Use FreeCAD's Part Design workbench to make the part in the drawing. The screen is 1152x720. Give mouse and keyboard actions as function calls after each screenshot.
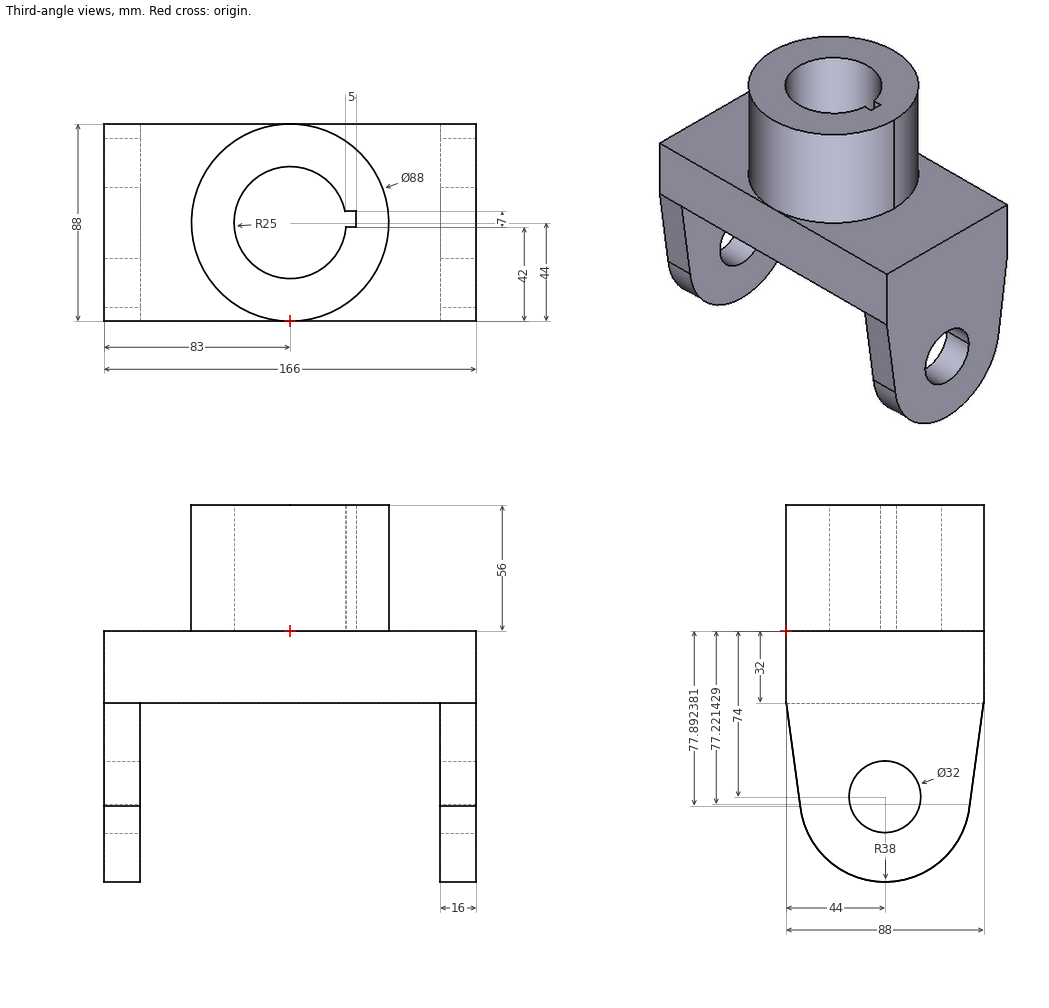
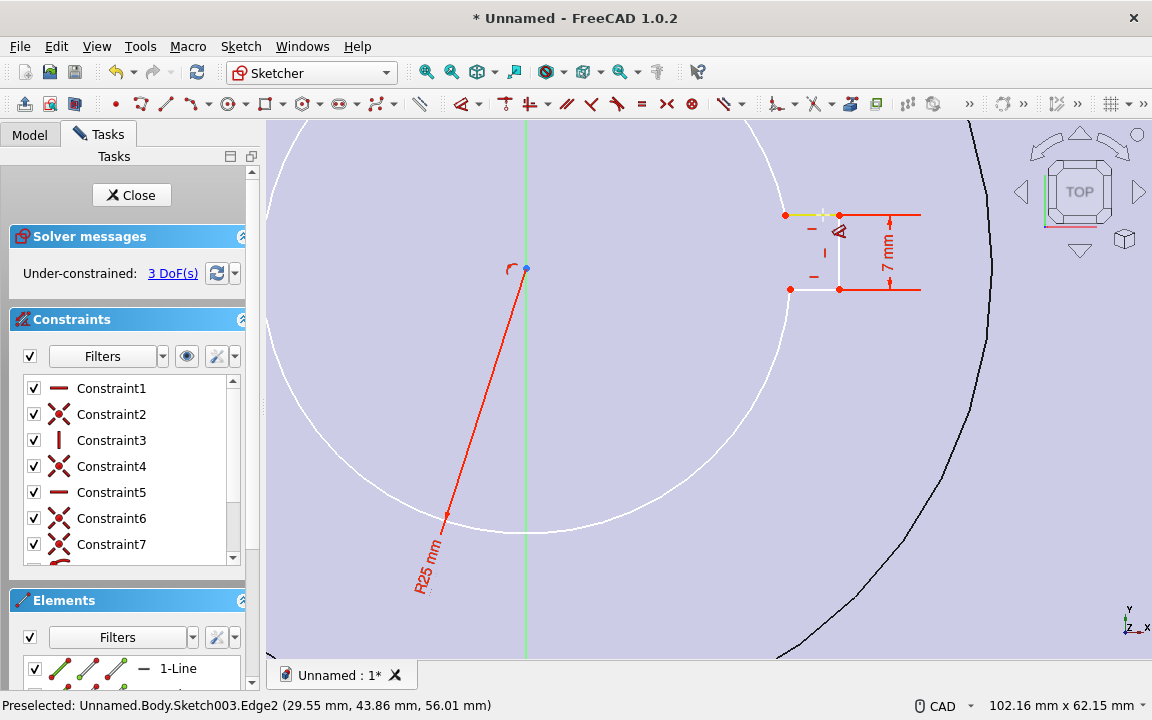
click(823, 215)
click(812, 181)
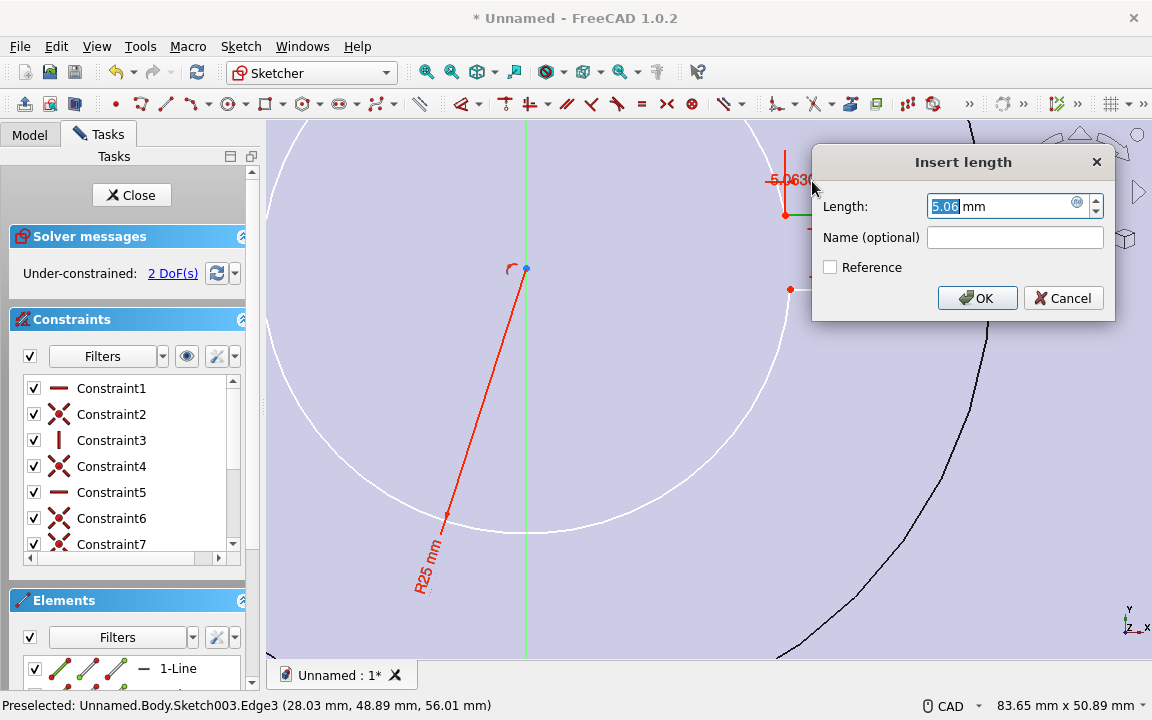
text(5)
key(Return)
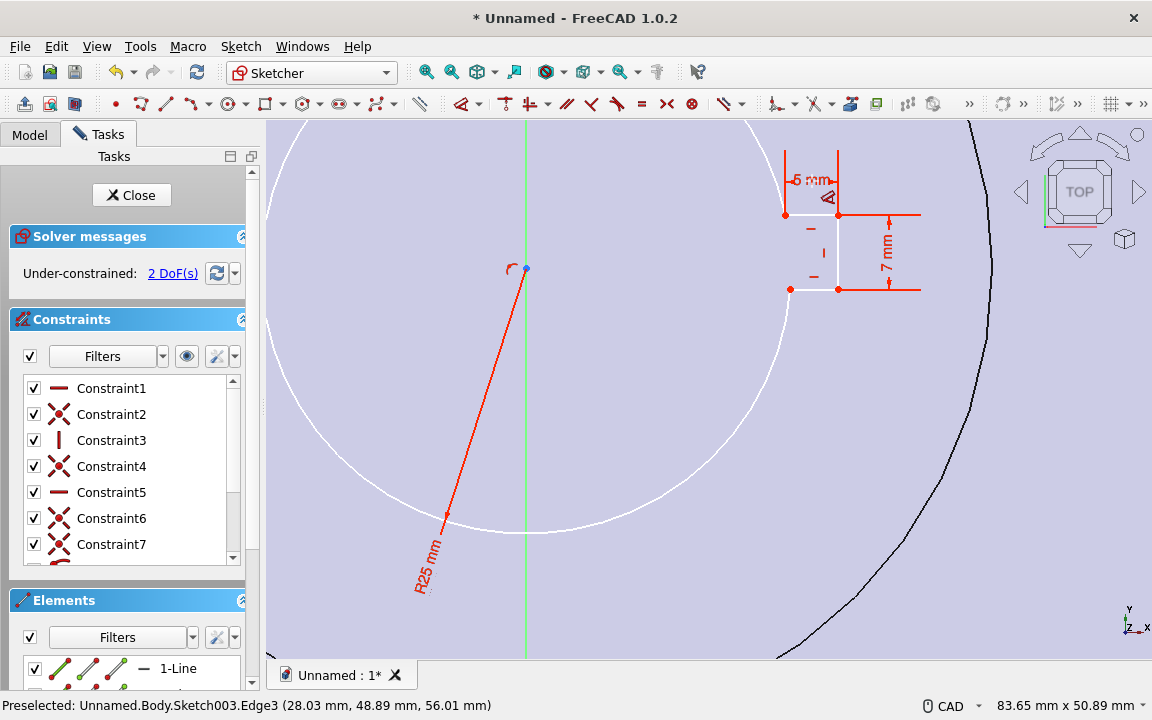
click(790, 290)
click(824, 460)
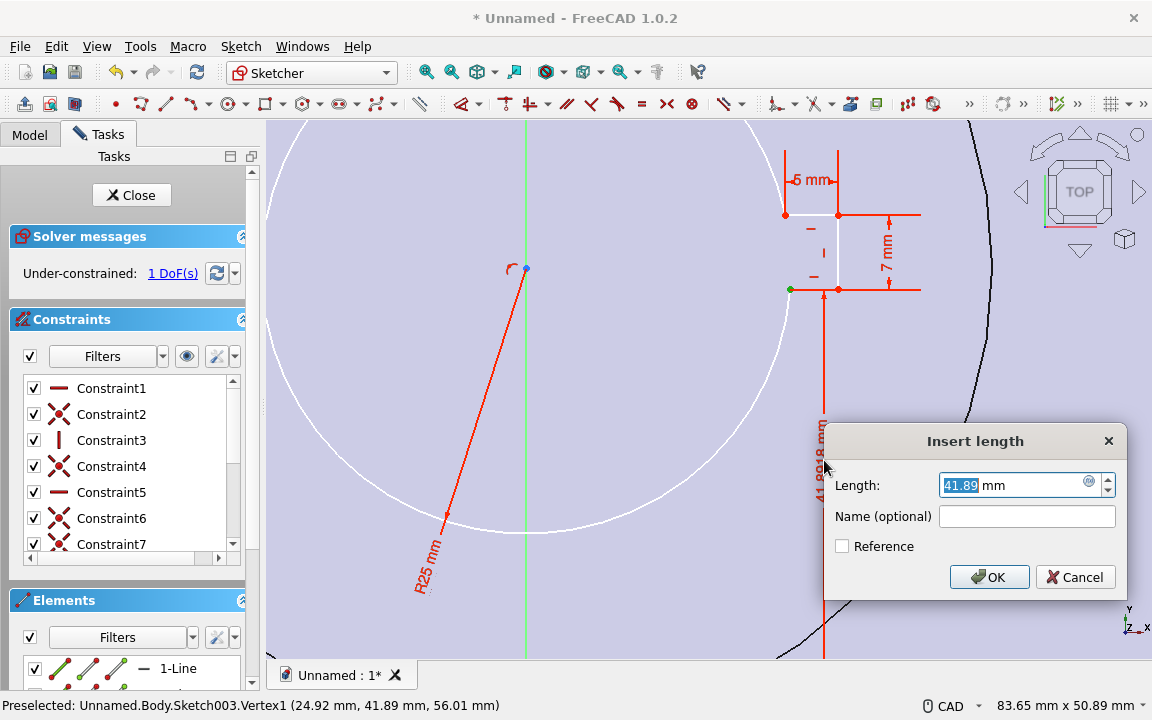
text(42)
key(Return)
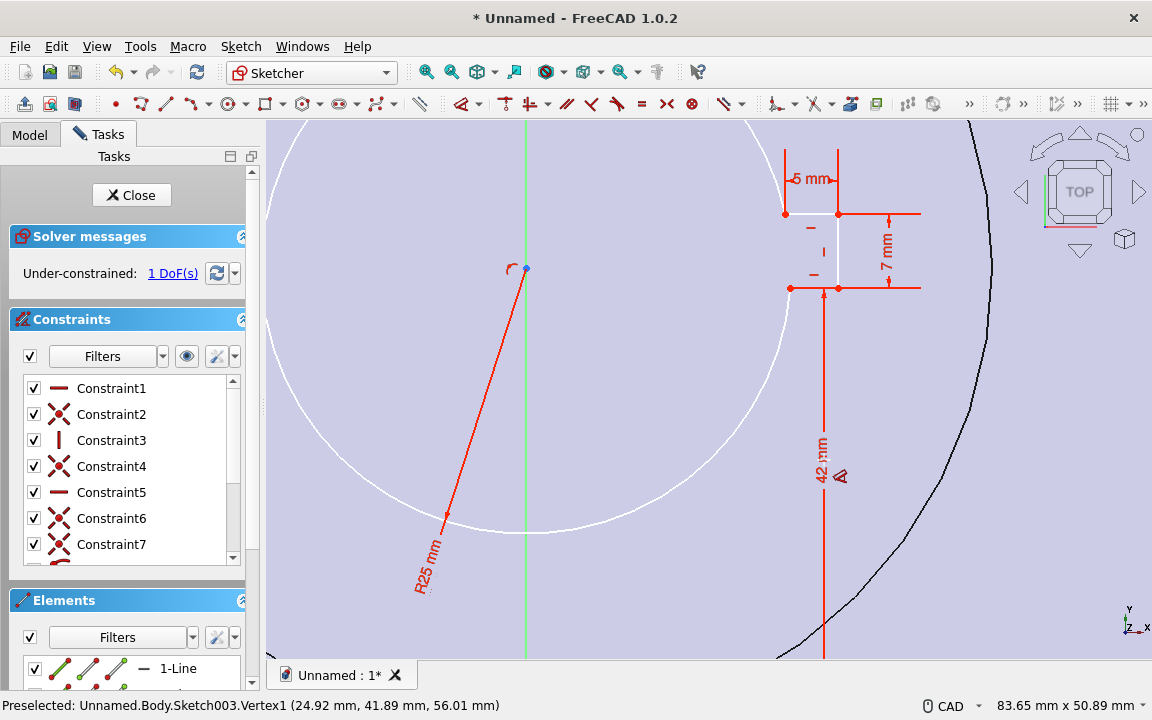
click(526, 269)
click(492, 450)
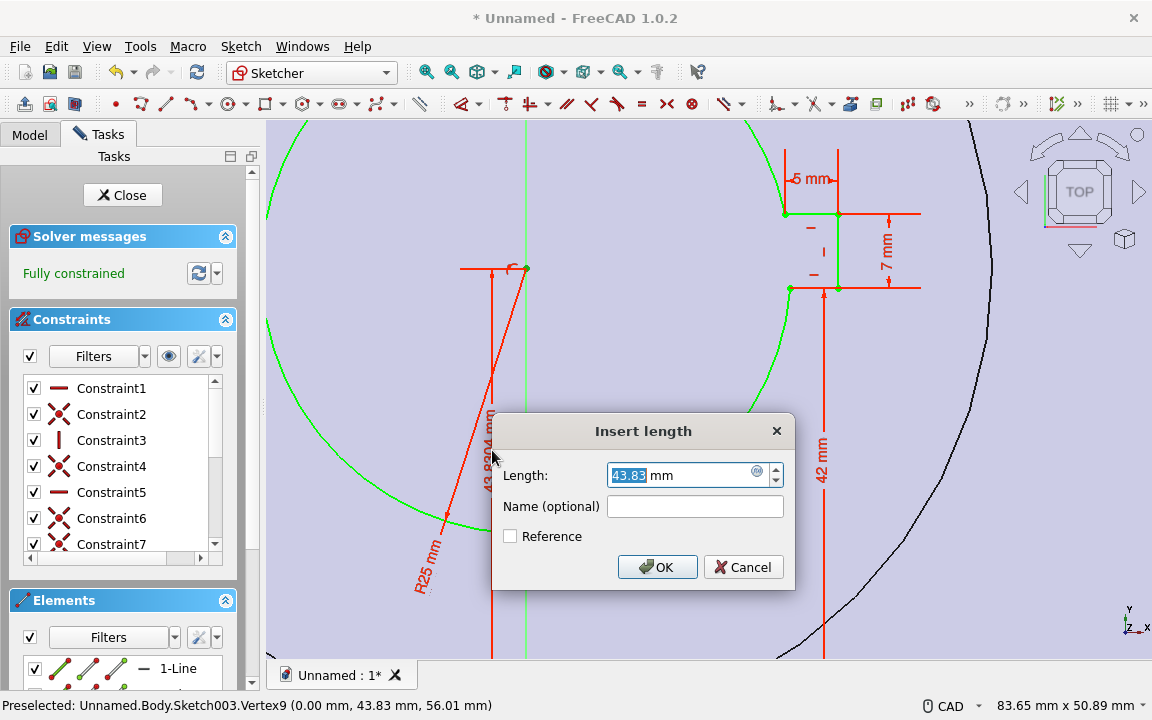
text(44)
key(Return)
key(Escape)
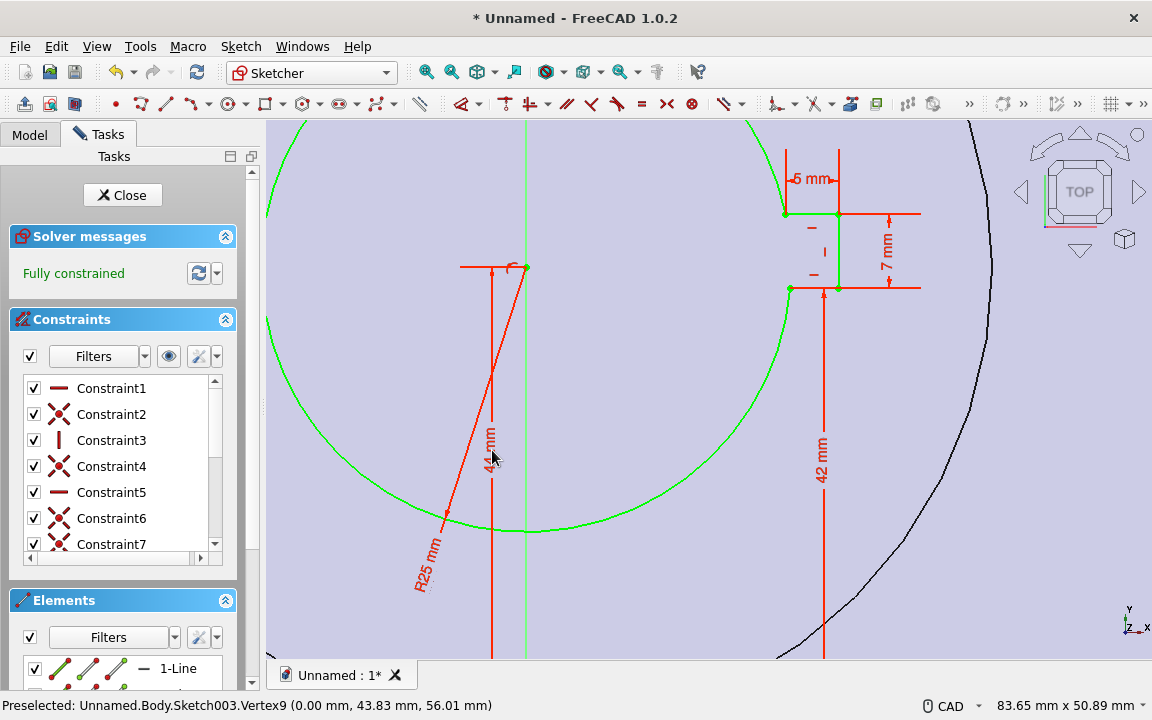
click(123, 195)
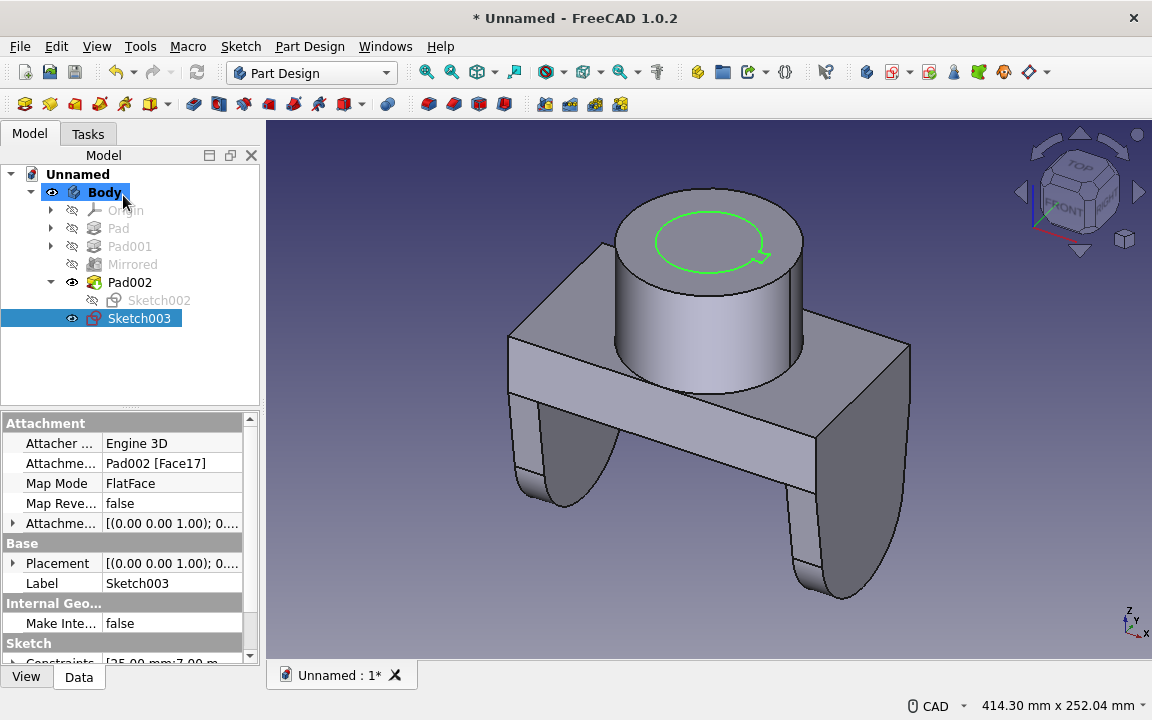
click(194, 104)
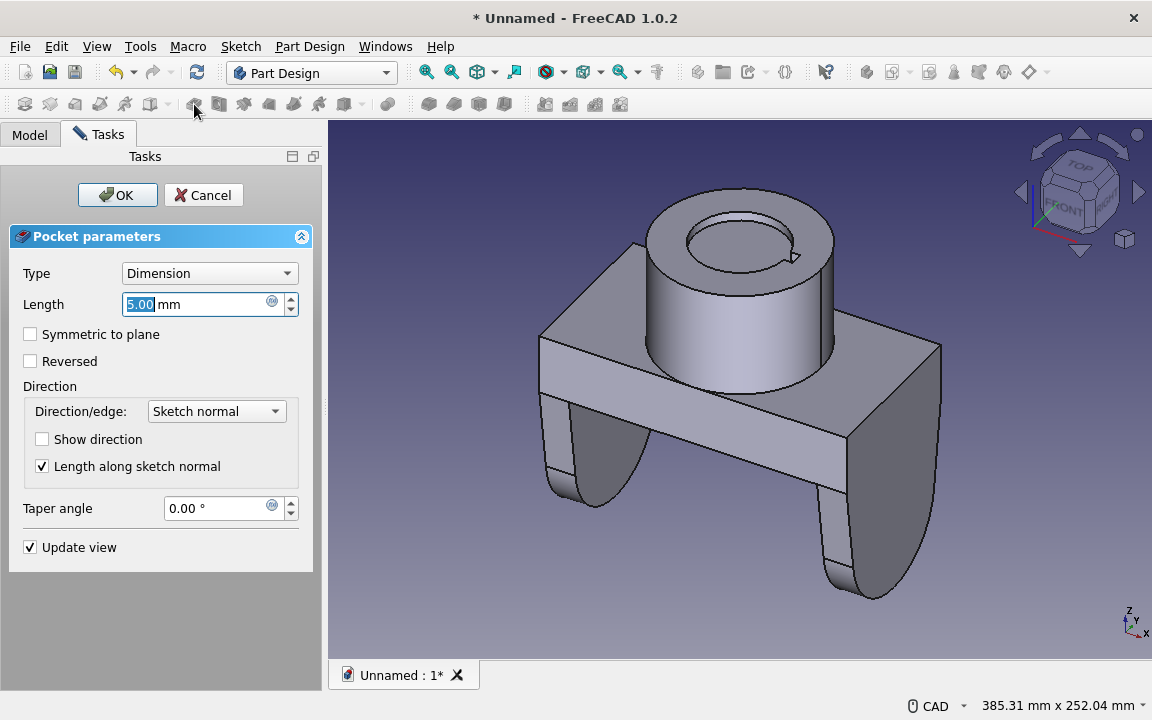
text(56)
key(Tab)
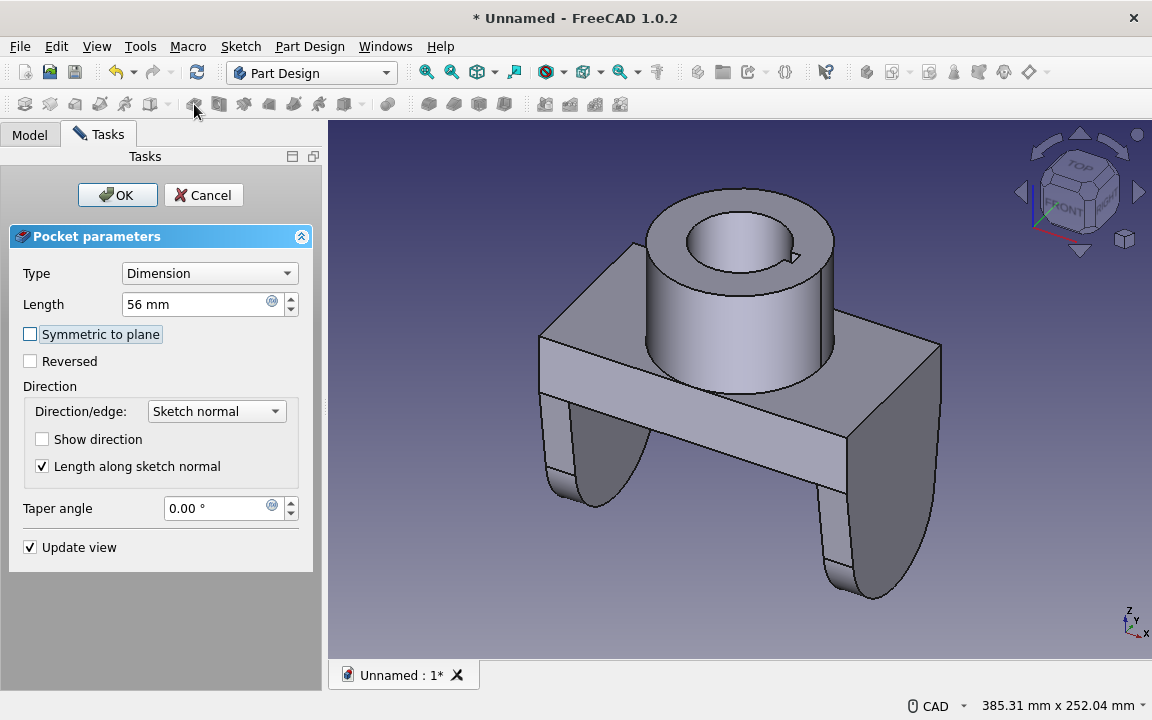
click(118, 195)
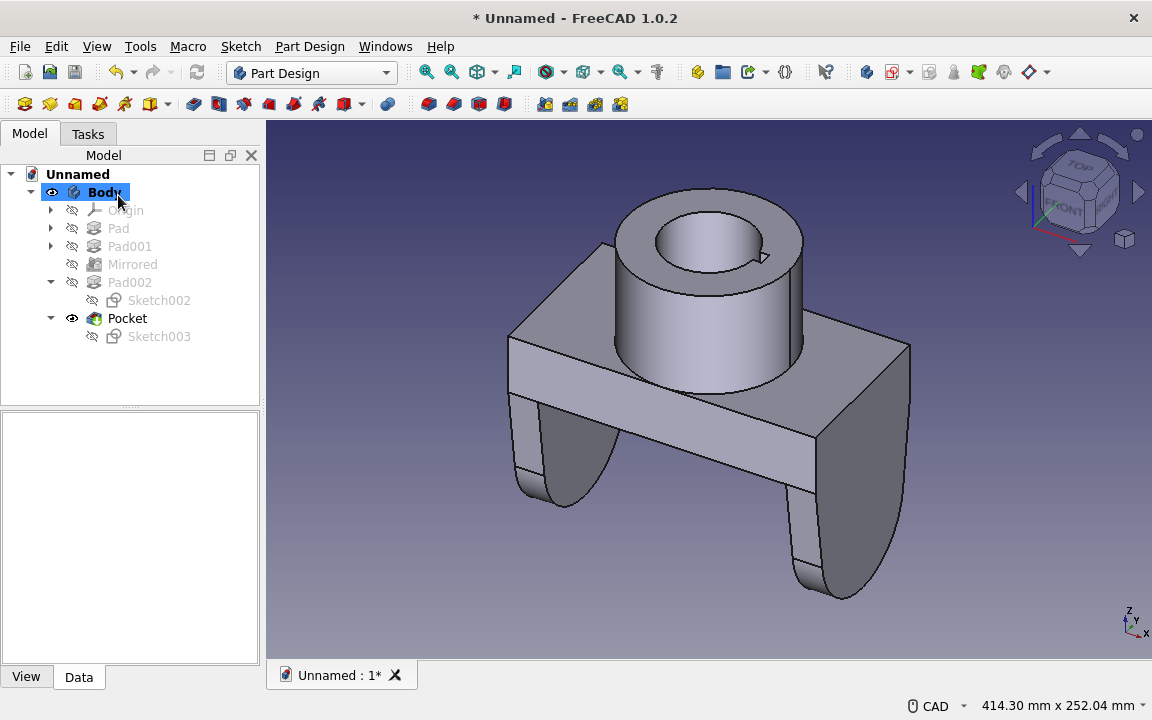
click(863, 488)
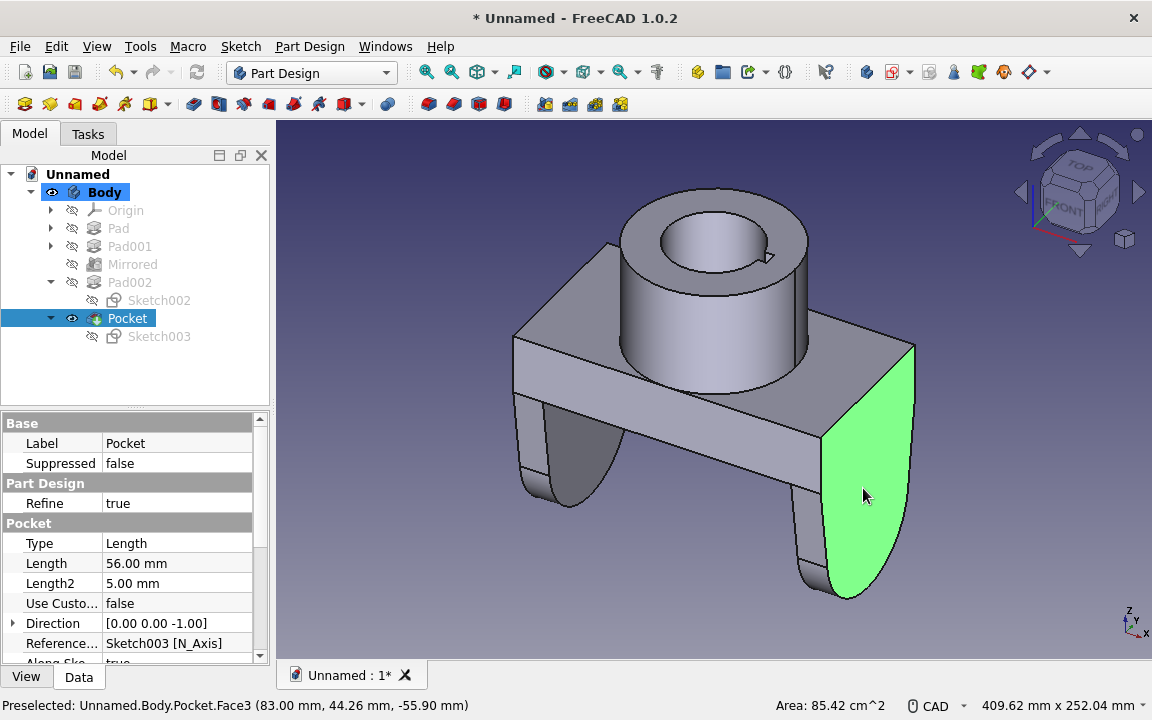
click(892, 72)